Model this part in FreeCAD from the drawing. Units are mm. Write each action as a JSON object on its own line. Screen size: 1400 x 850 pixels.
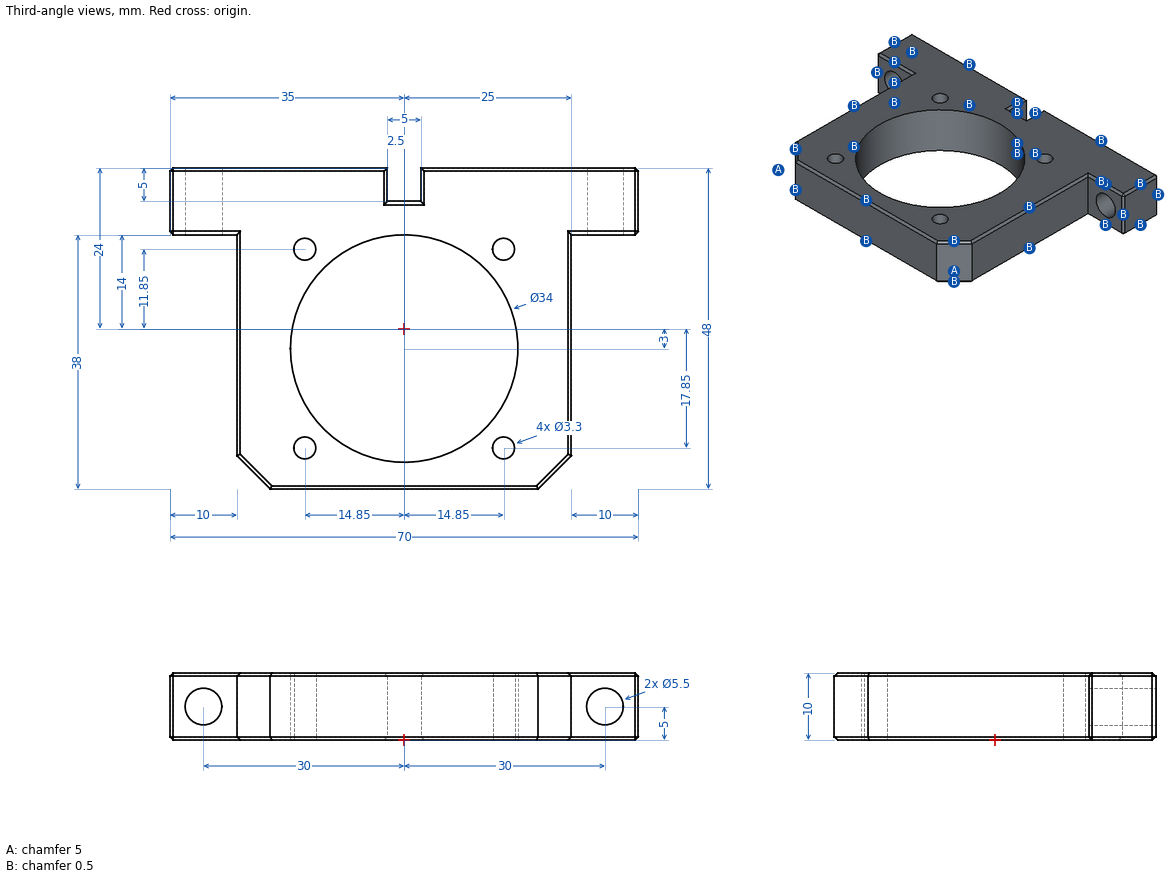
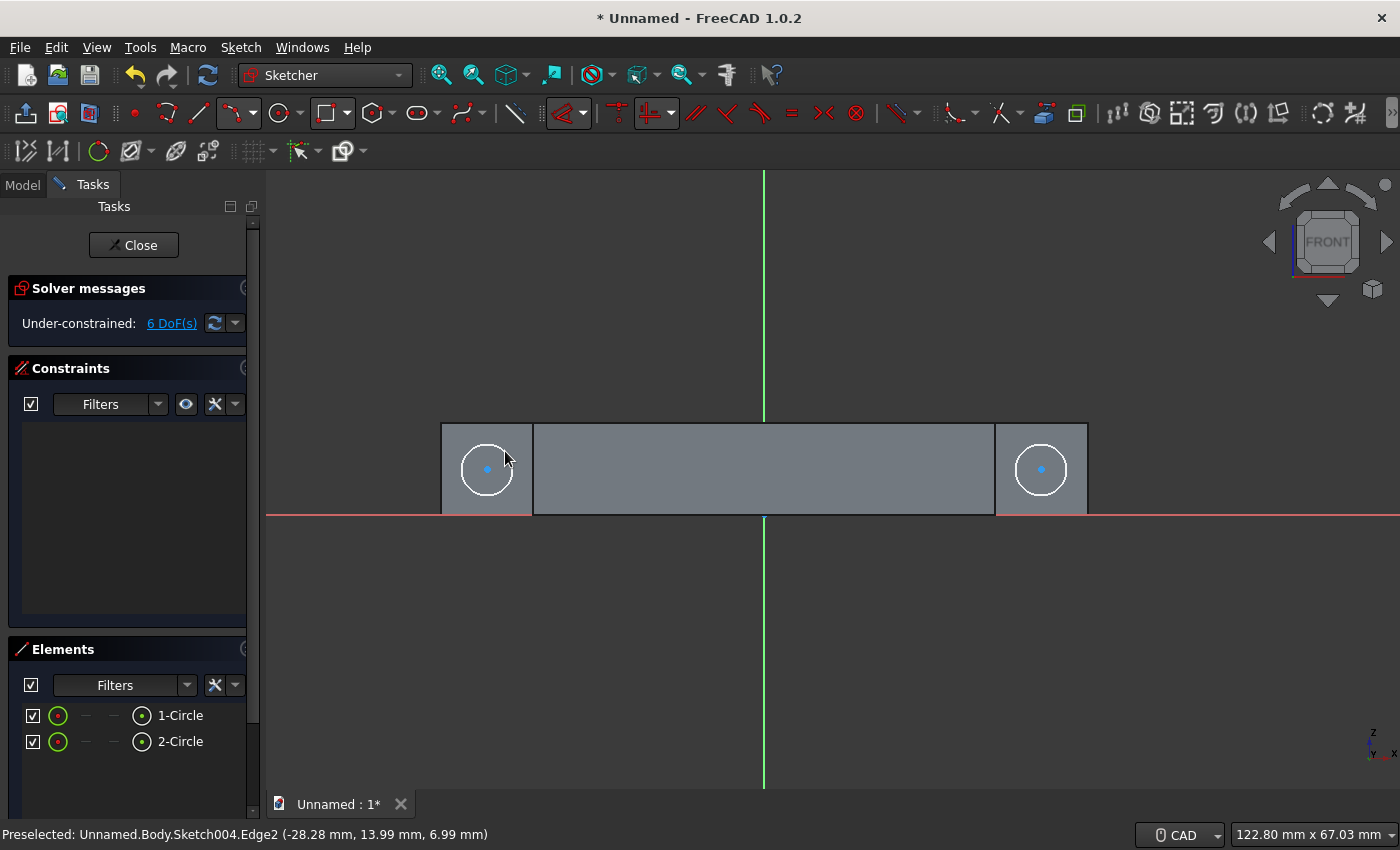
{"action": "left_click", "coordinate": [1059, 452]}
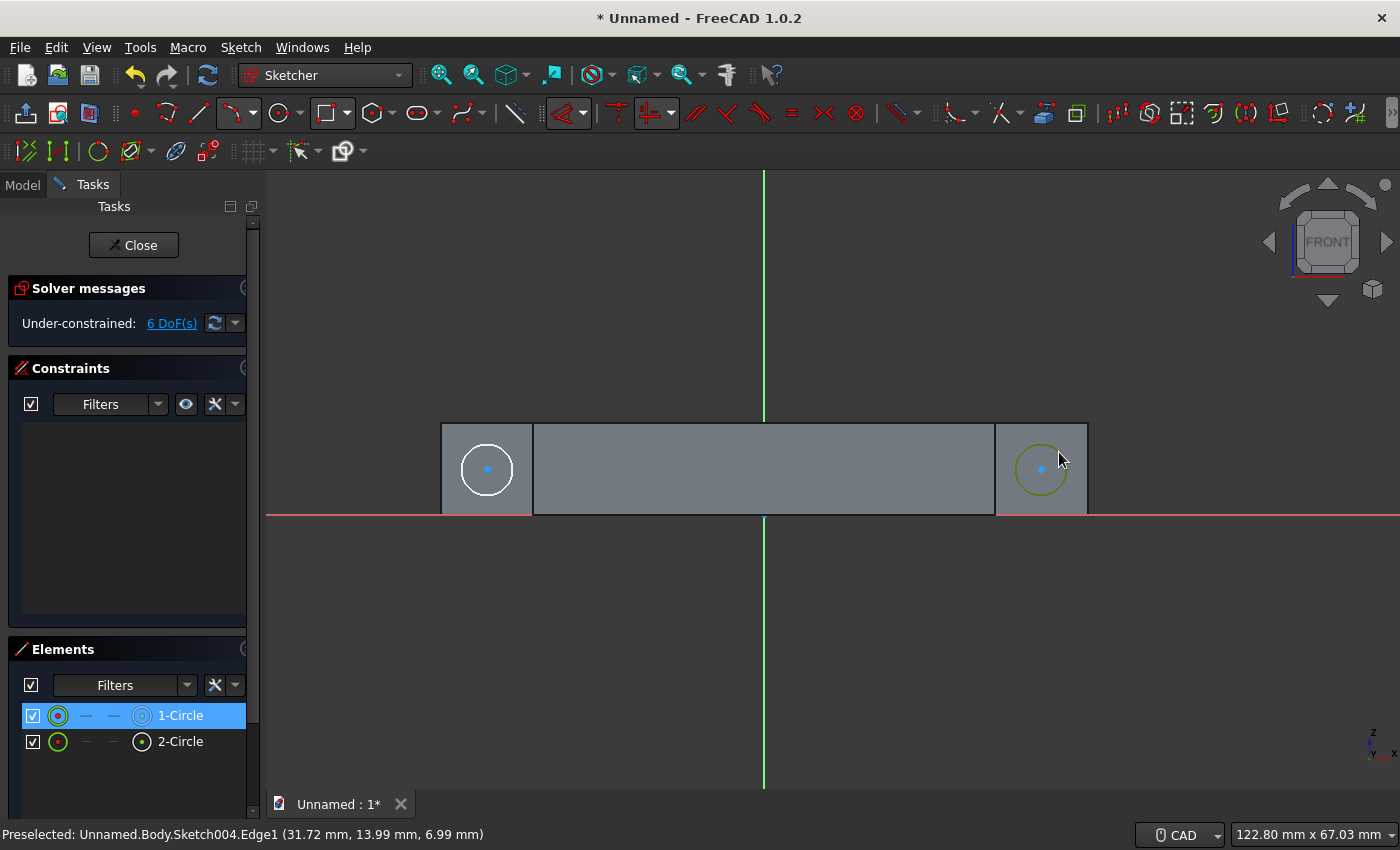
{"action": "left_click", "coordinate": [505, 452]}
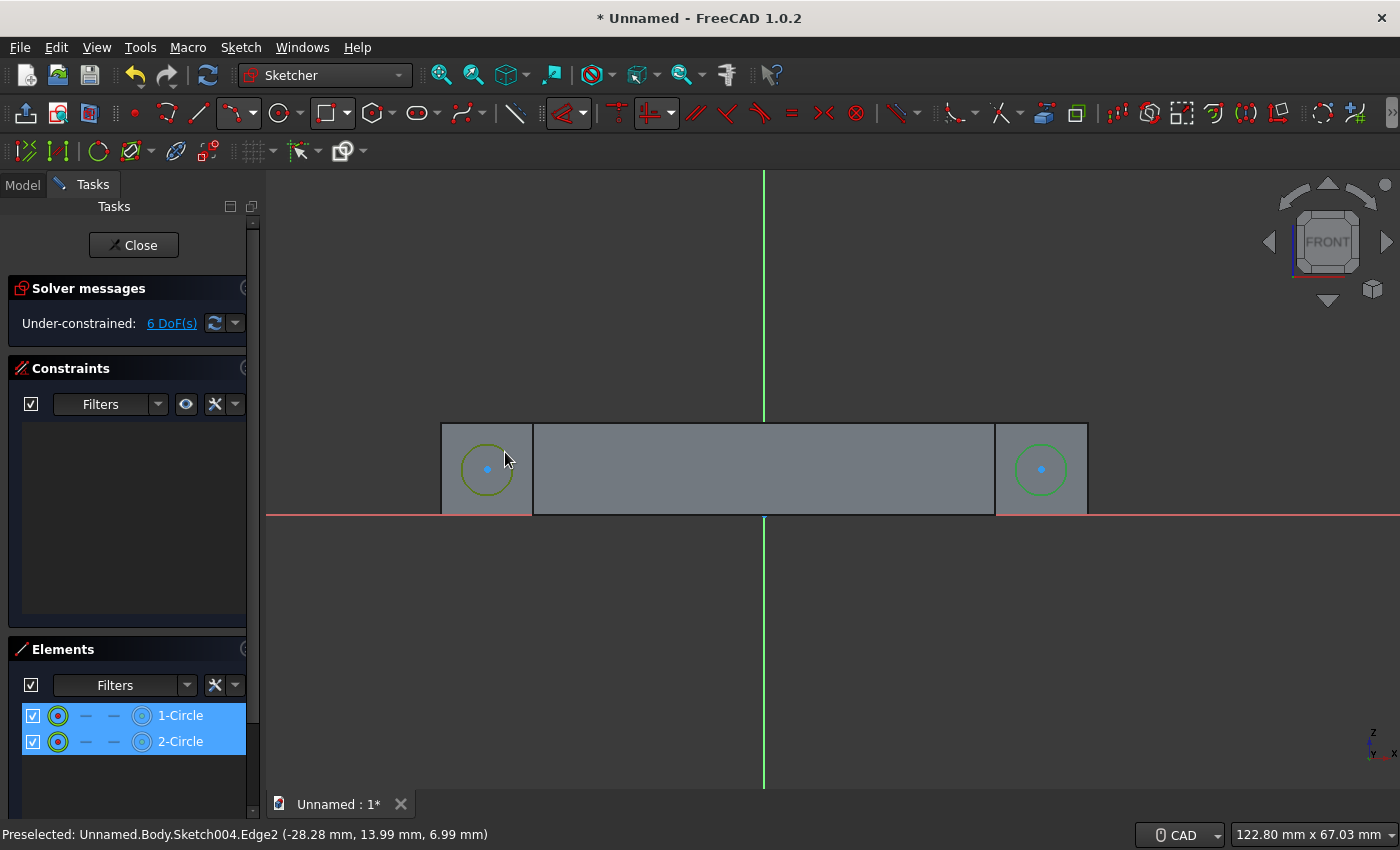
{"action": "key", "text": "e"}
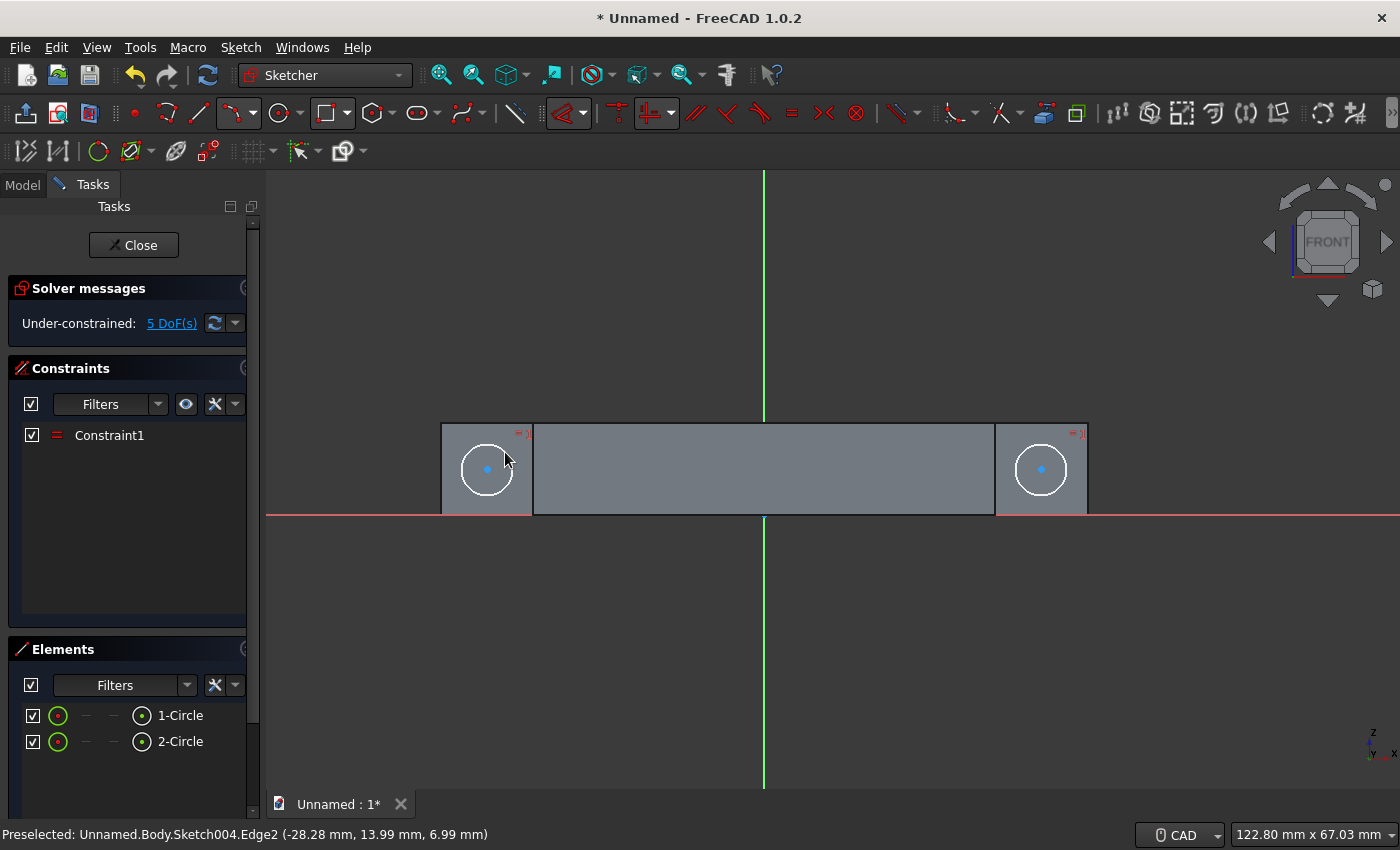
{"action": "left_click", "coordinate": [1041, 470]}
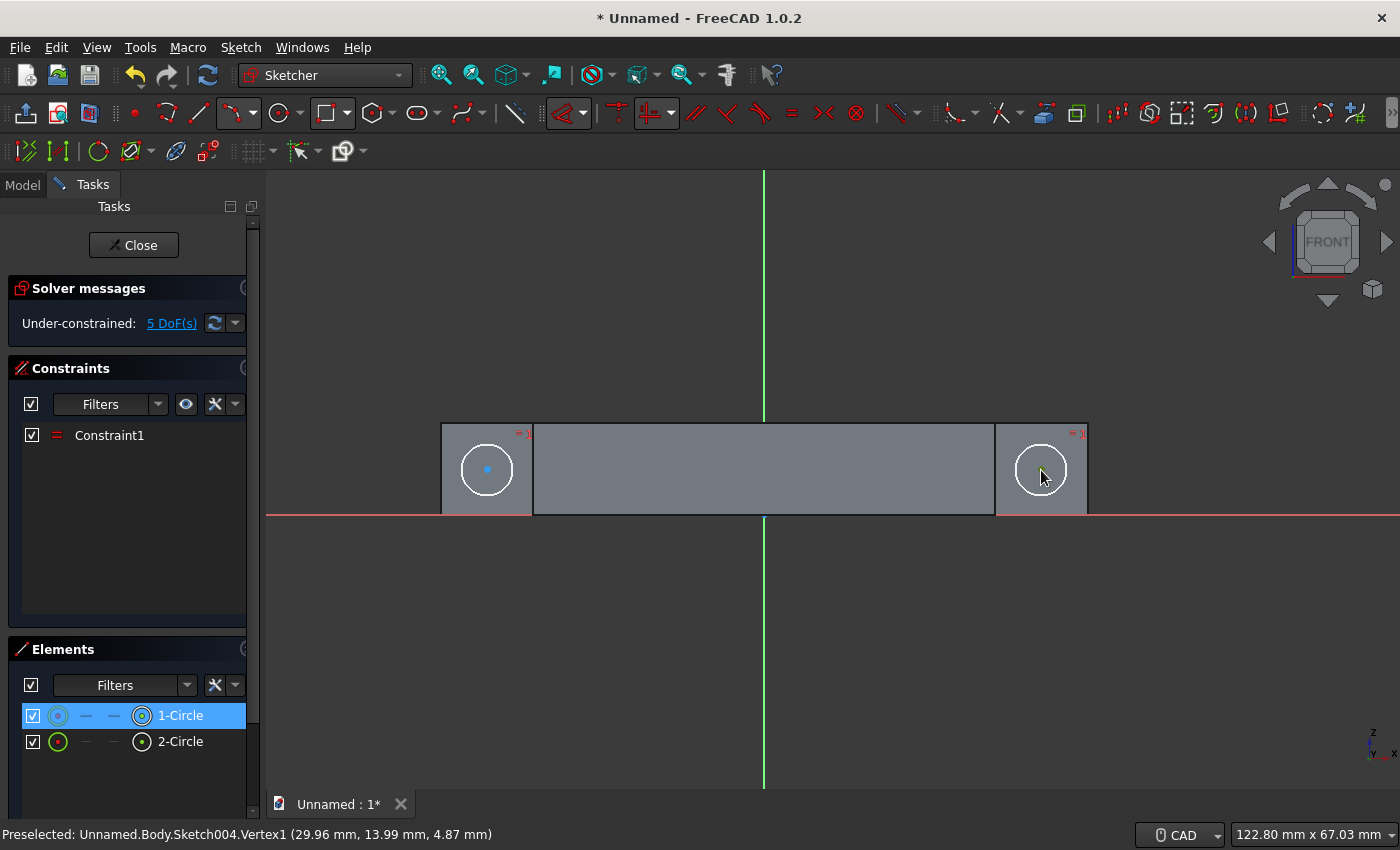
{"action": "left_click", "coordinate": [487, 470]}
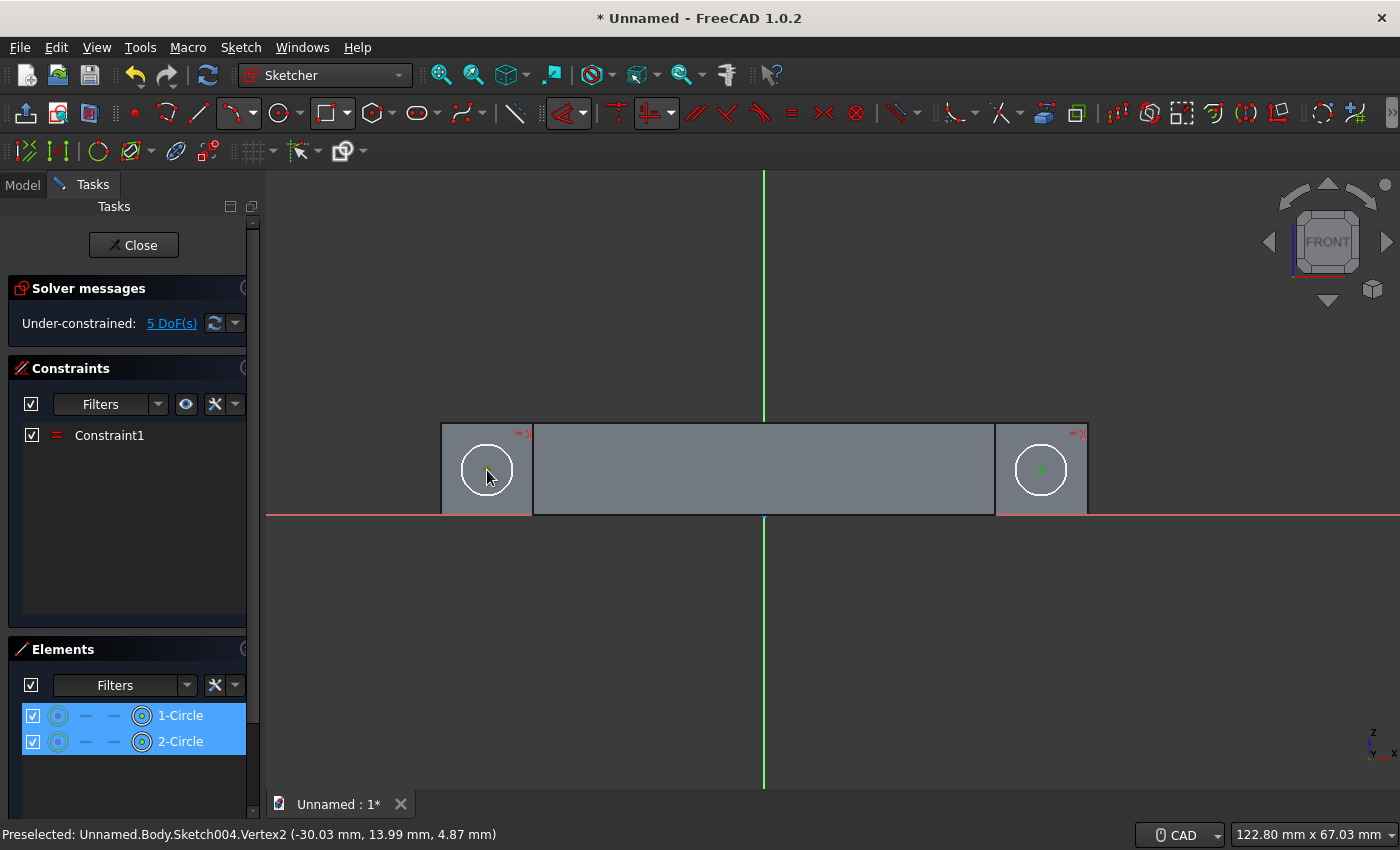
{"action": "left_click", "coordinate": [674, 114]}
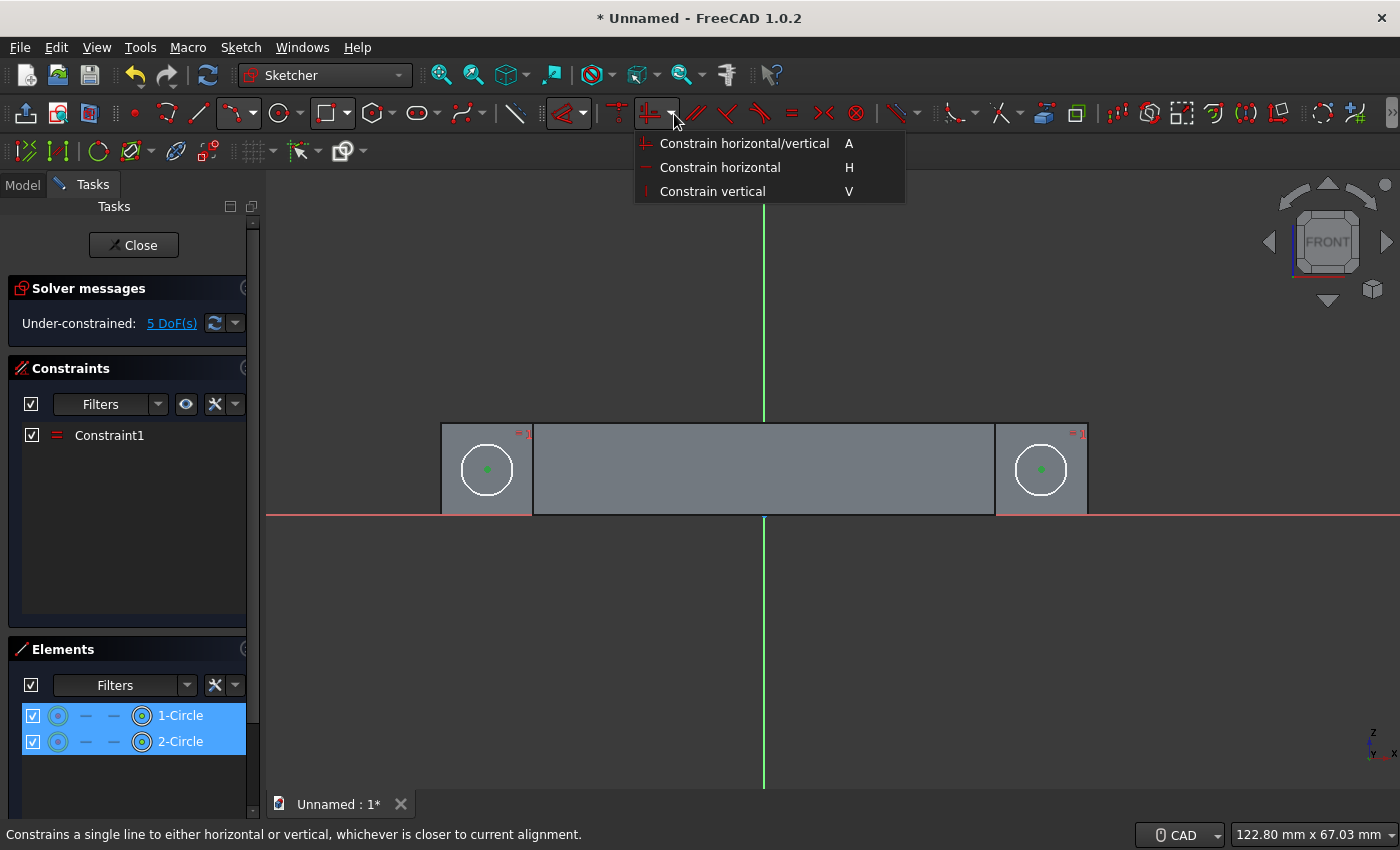
{"action": "left_click", "coordinate": [770, 167]}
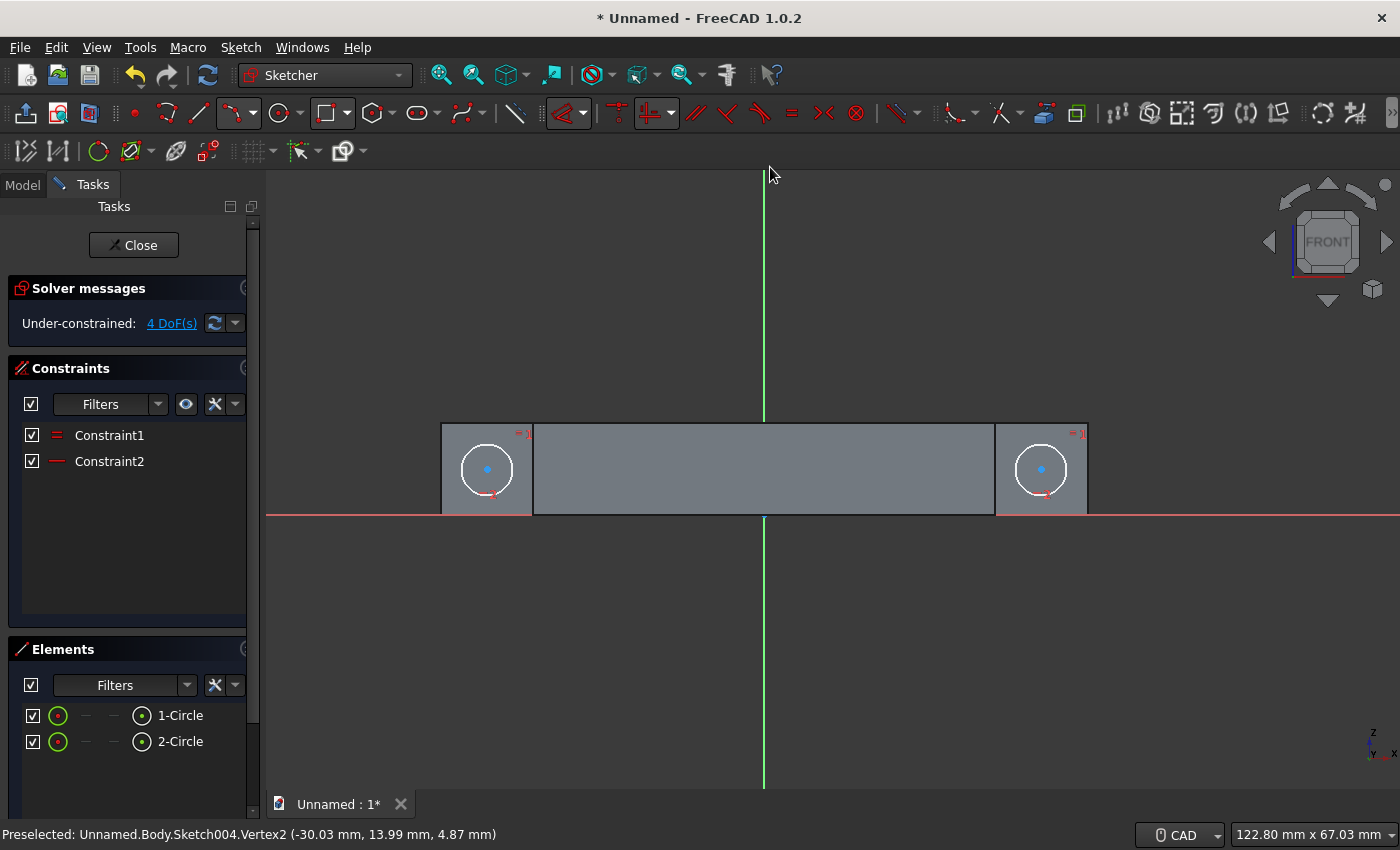
{"action": "left_click", "coordinate": [1059, 452]}